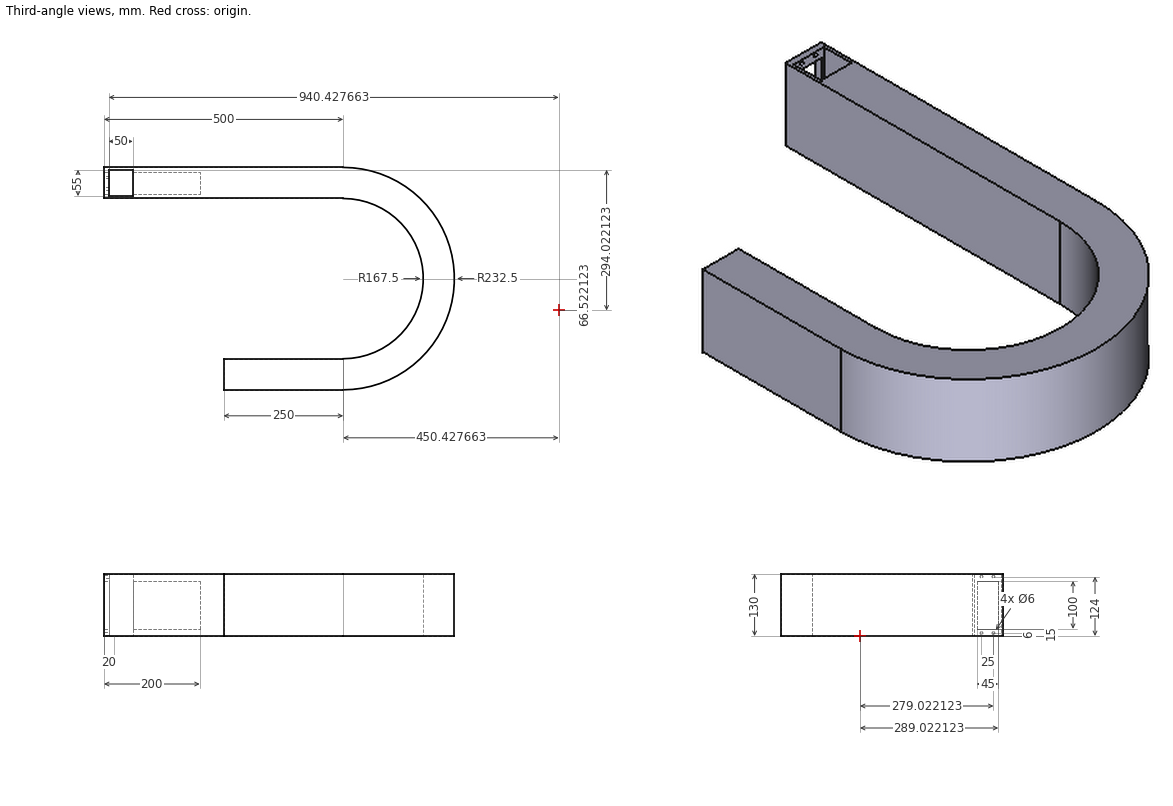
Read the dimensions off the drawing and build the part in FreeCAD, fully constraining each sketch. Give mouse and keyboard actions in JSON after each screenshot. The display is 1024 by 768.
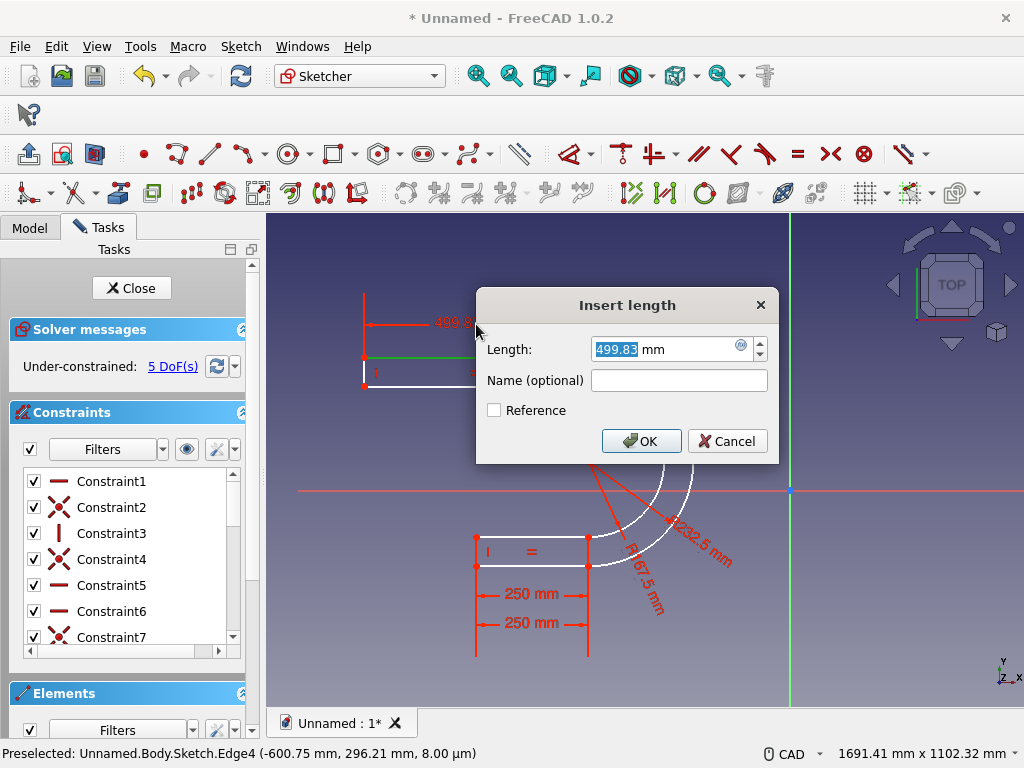
{"action": "type", "text": "500"}
{"action": "key", "text": "Return"}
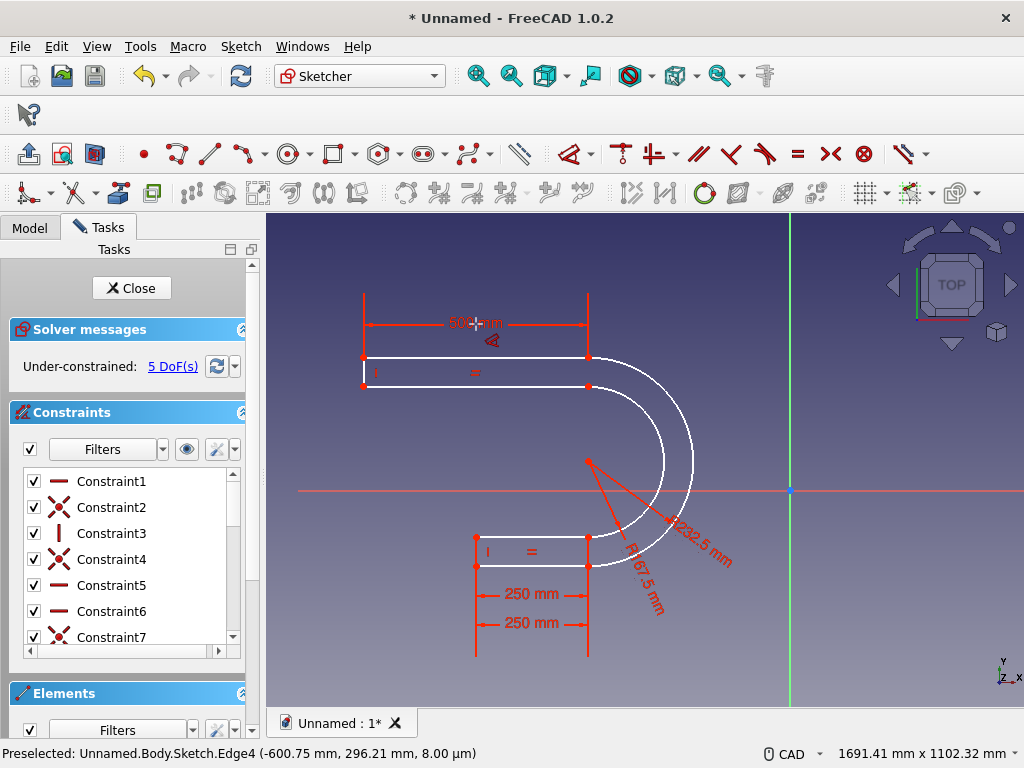
{"action": "left_click", "coordinate": [431, 387]}
{"action": "left_click", "coordinate": [476, 421]}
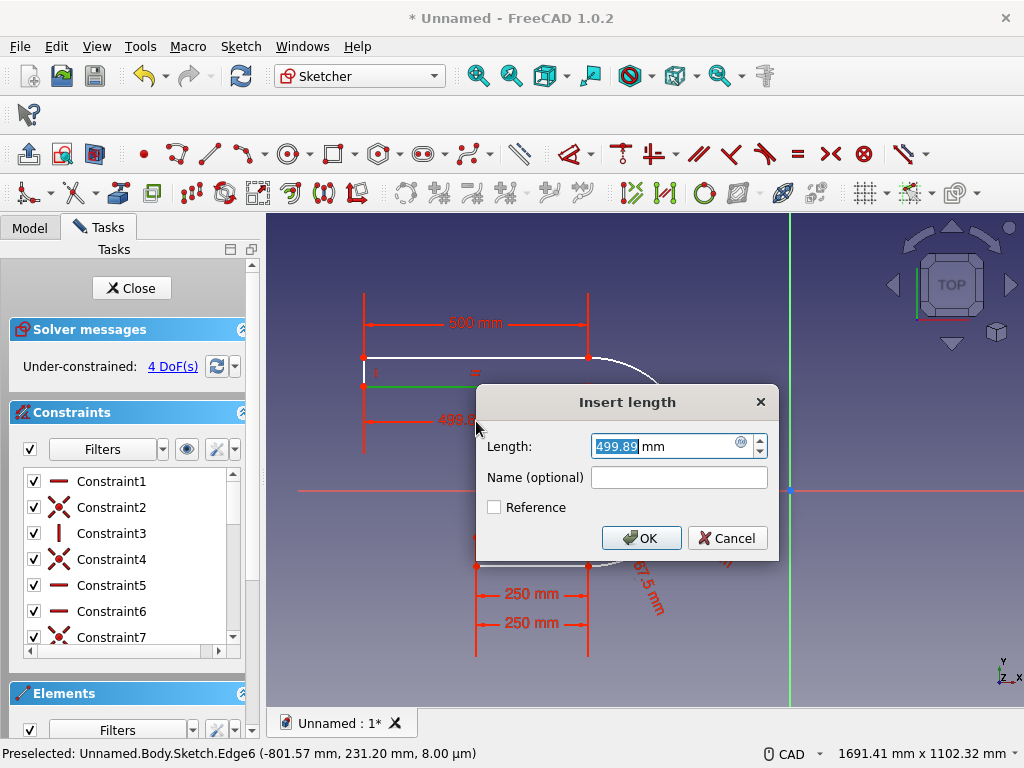
{"action": "type", "text": "500"}
{"action": "key", "text": "Return"}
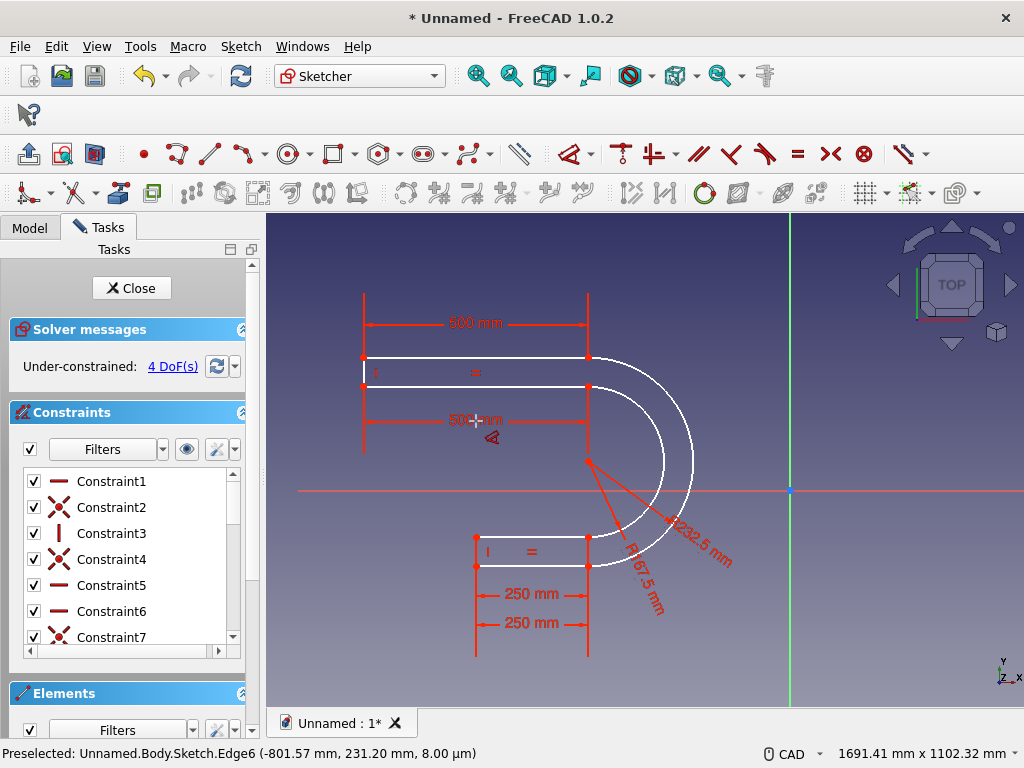
{"action": "scroll", "coordinate": [589, 462], "scroll_direction": "up", "scroll_amount": 2}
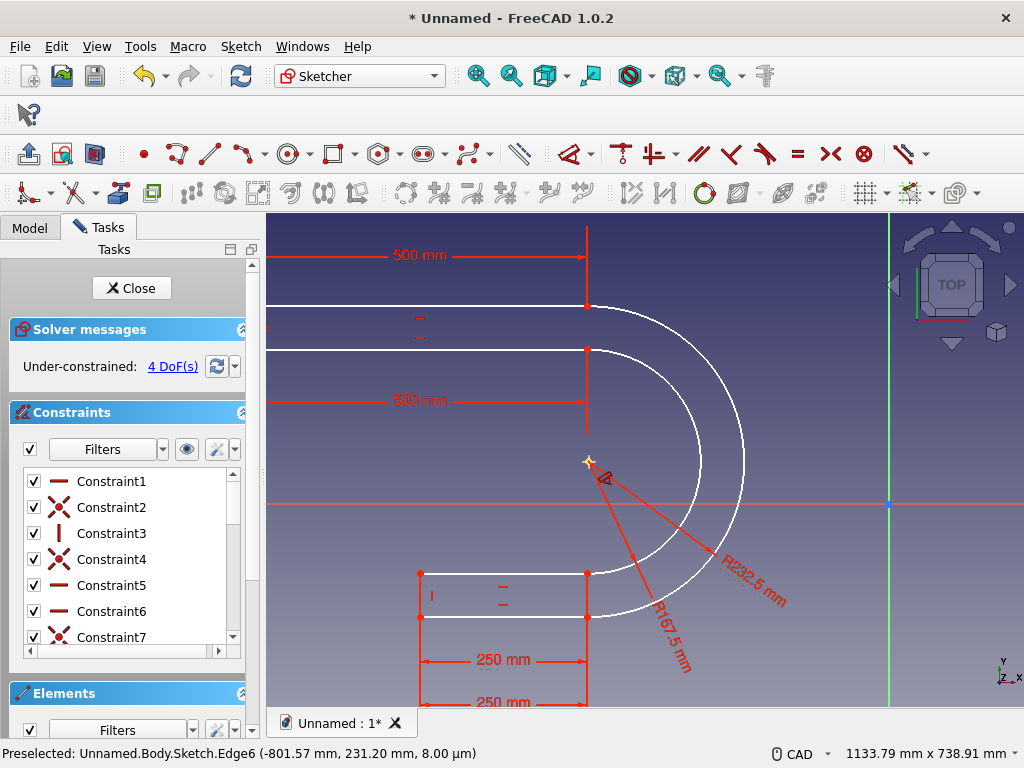
{"action": "left_click", "coordinate": [589, 462]}
{"action": "left_click", "coordinate": [555, 483]}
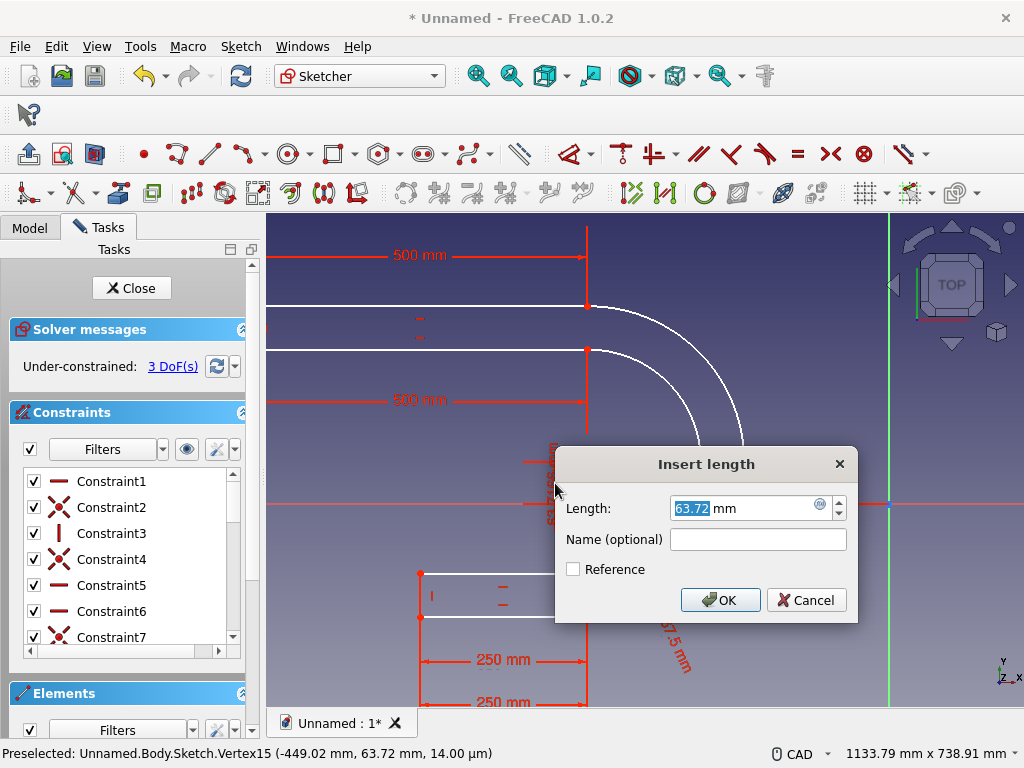
{"action": "type", "text": "66.522123"}
{"action": "key", "text": "Return"}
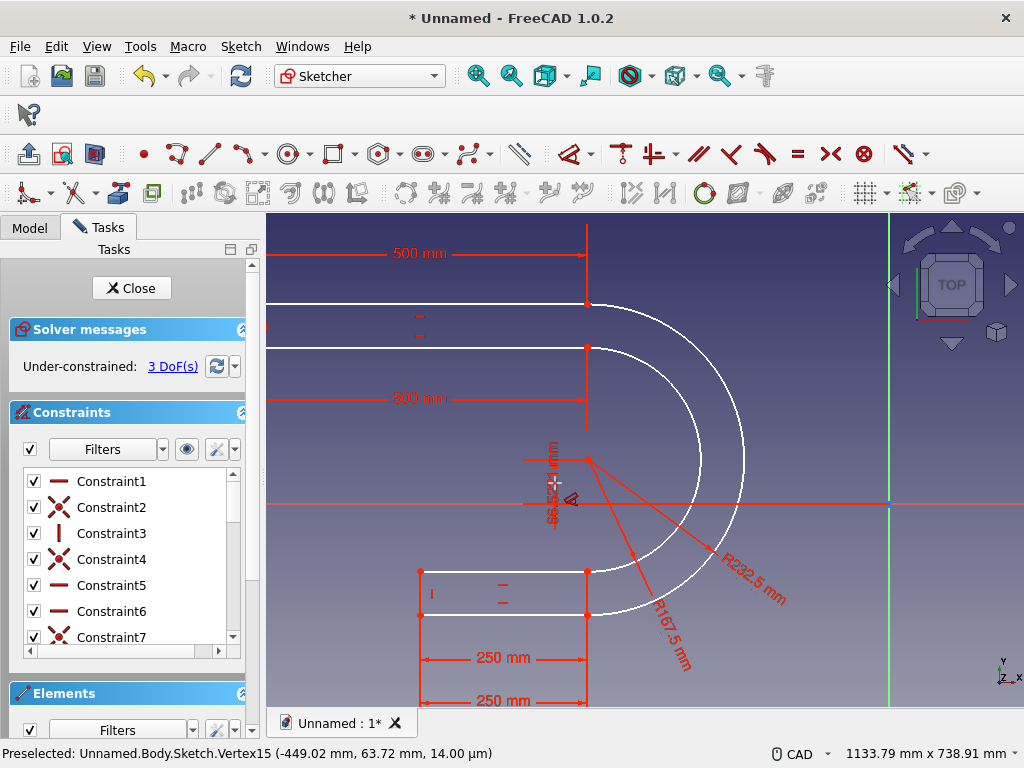
{"action": "left_click", "coordinate": [587, 572]}
{"action": "left_click", "coordinate": [723, 606]}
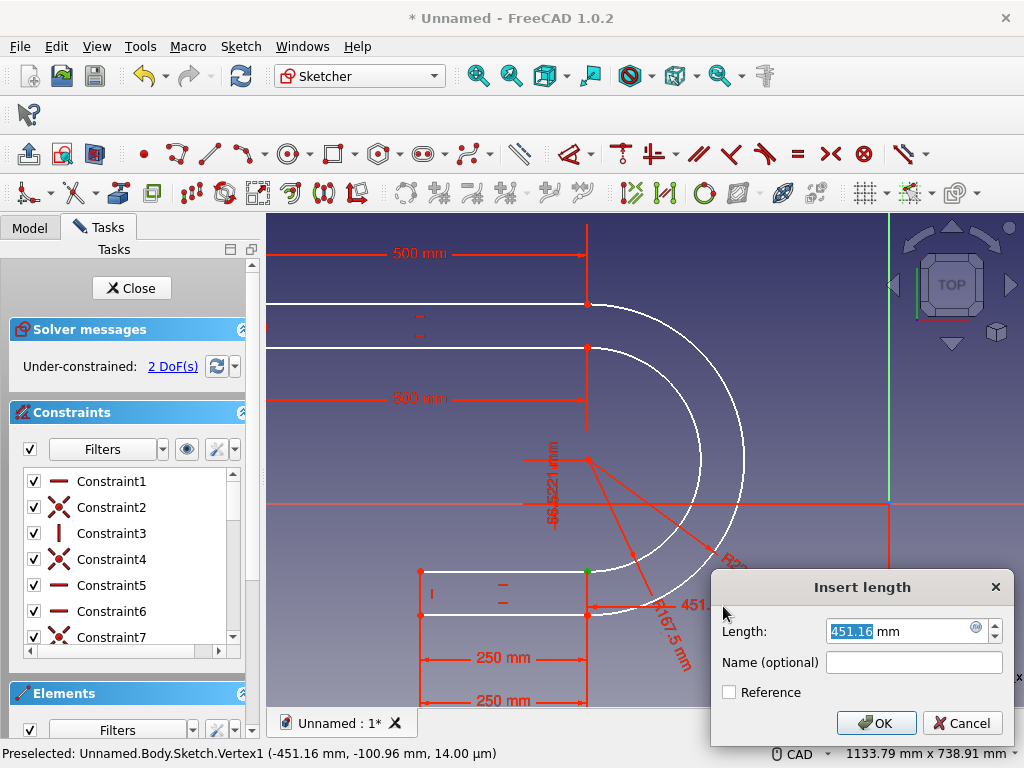
{"action": "type", "text": "450.427663"}
{"action": "key", "text": "Return"}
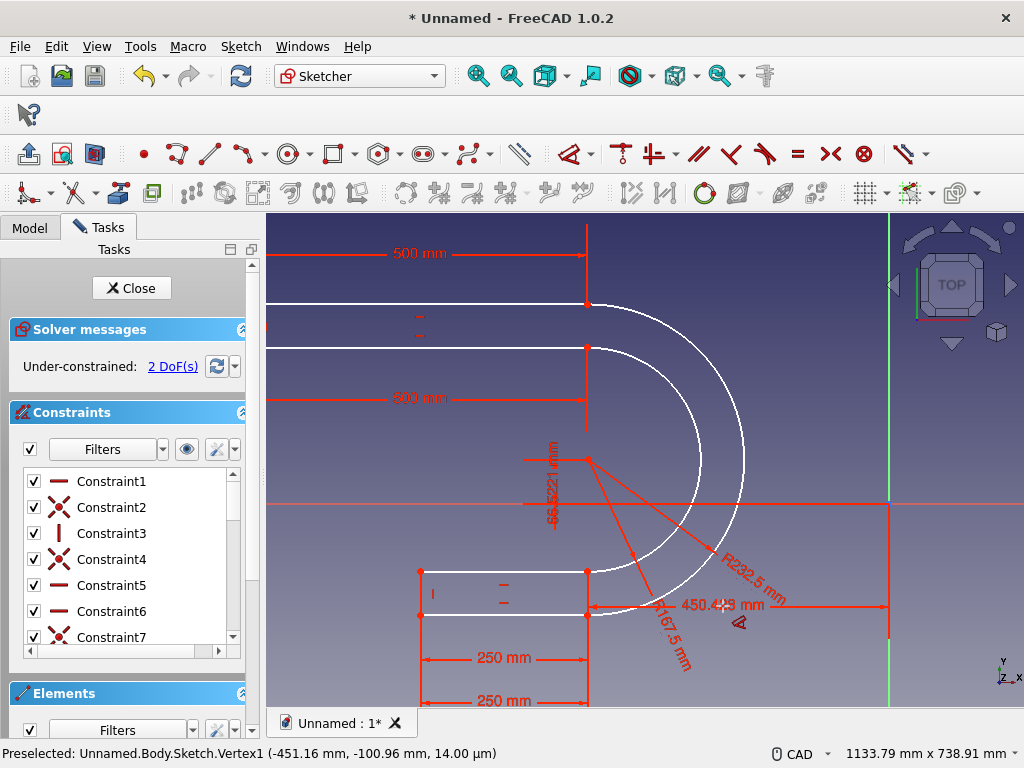
{"action": "left_click", "coordinate": [587, 304]}
{"action": "left_click", "coordinate": [723, 270]}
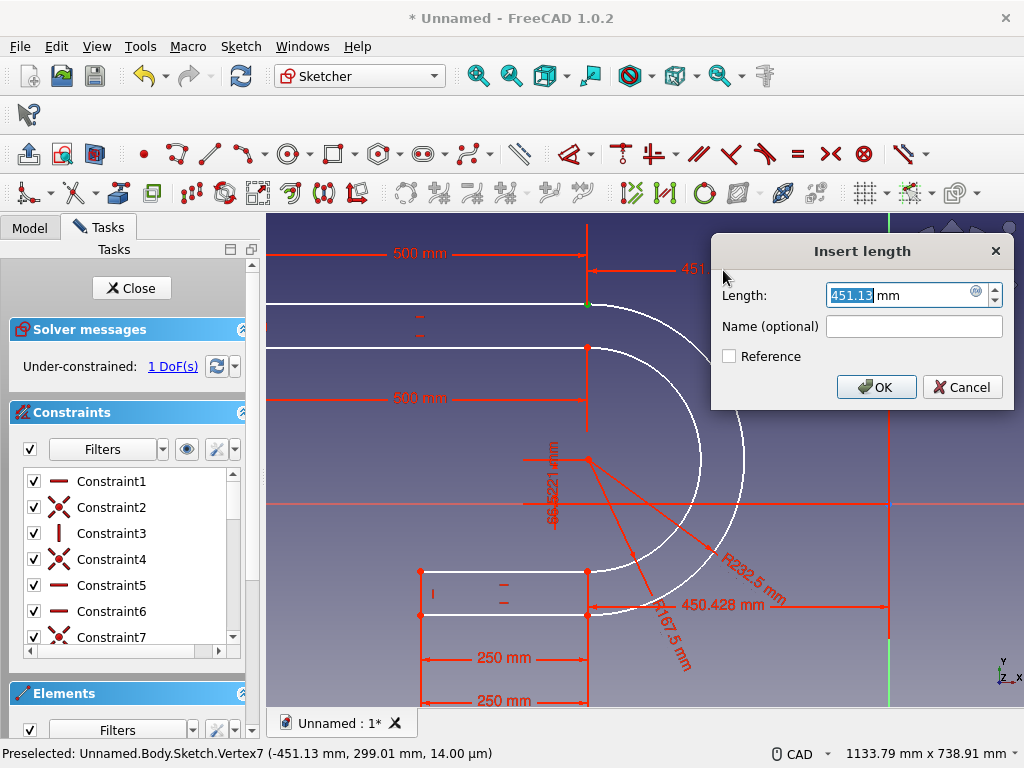
{"action": "type", "text": "450.427663"}
{"action": "key", "text": "Return"}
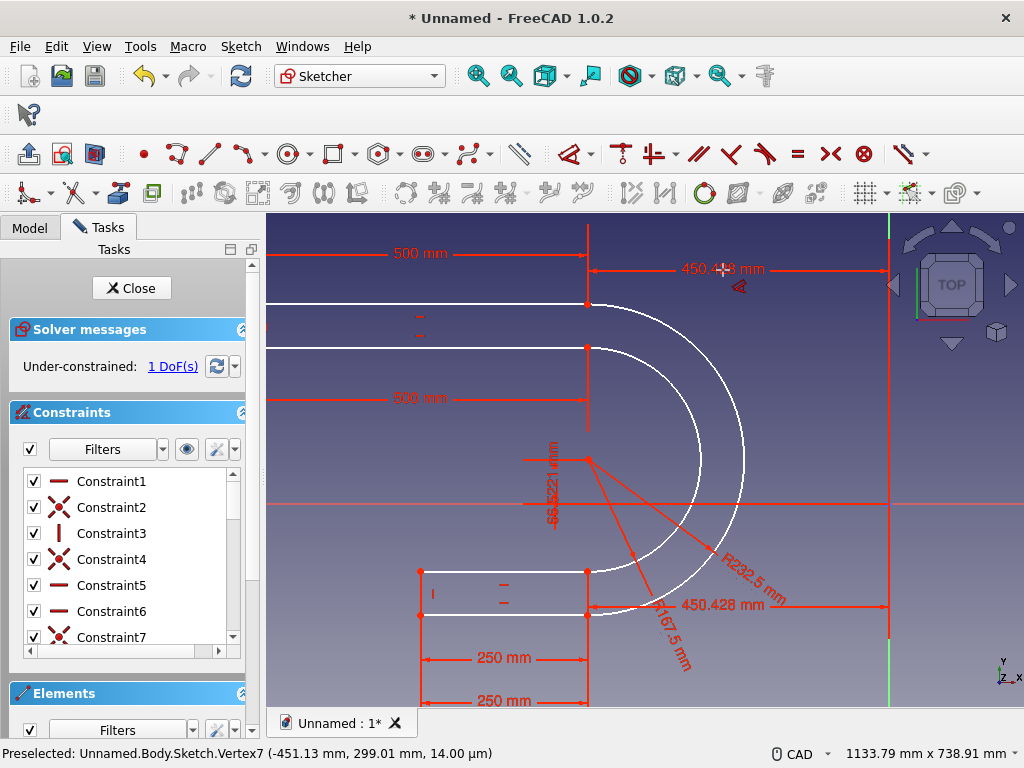
{"action": "left_click", "coordinate": [589, 460]}
{"action": "left_click", "coordinate": [786, 538]}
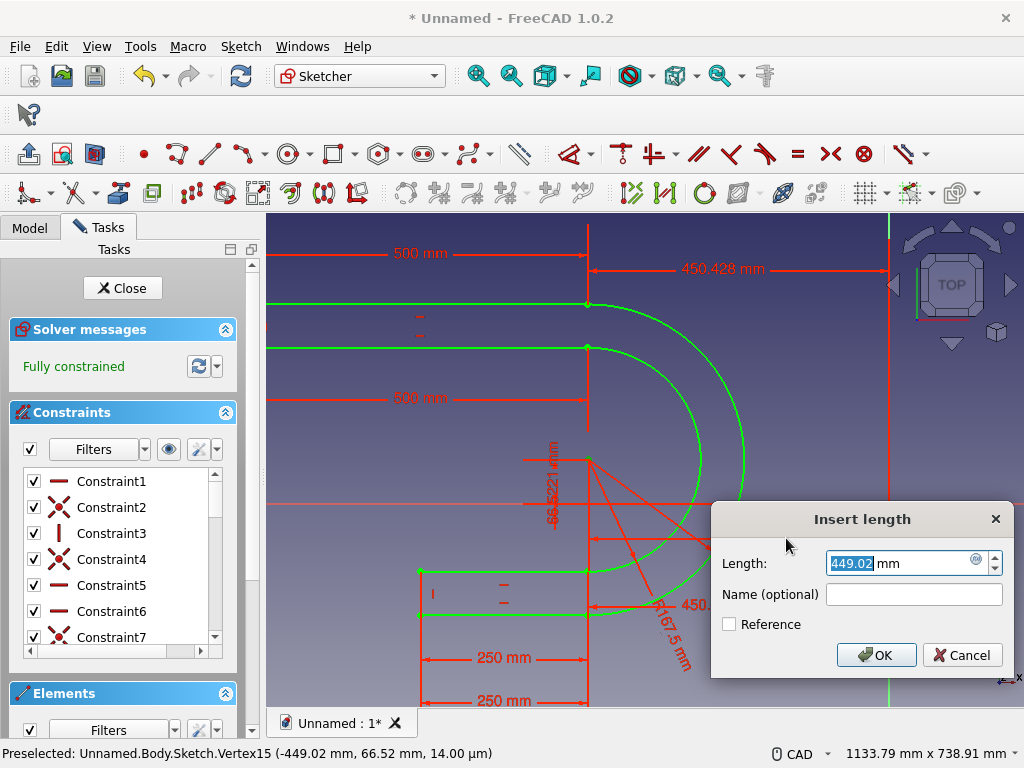
{"action": "type", "text": "450.427663"}
{"action": "key", "text": "Return"}
{"action": "key", "text": "Escape"}